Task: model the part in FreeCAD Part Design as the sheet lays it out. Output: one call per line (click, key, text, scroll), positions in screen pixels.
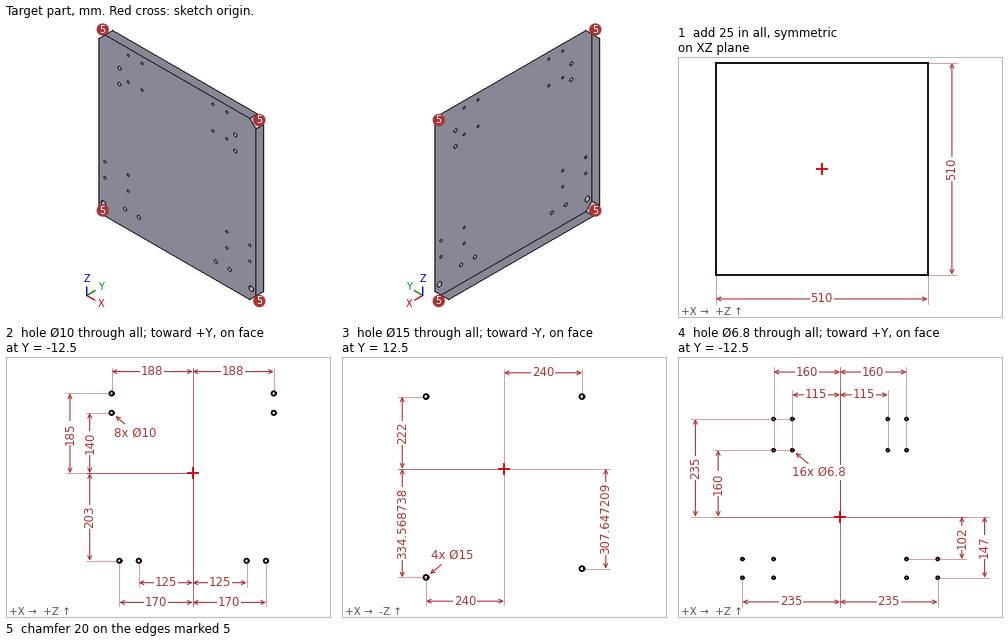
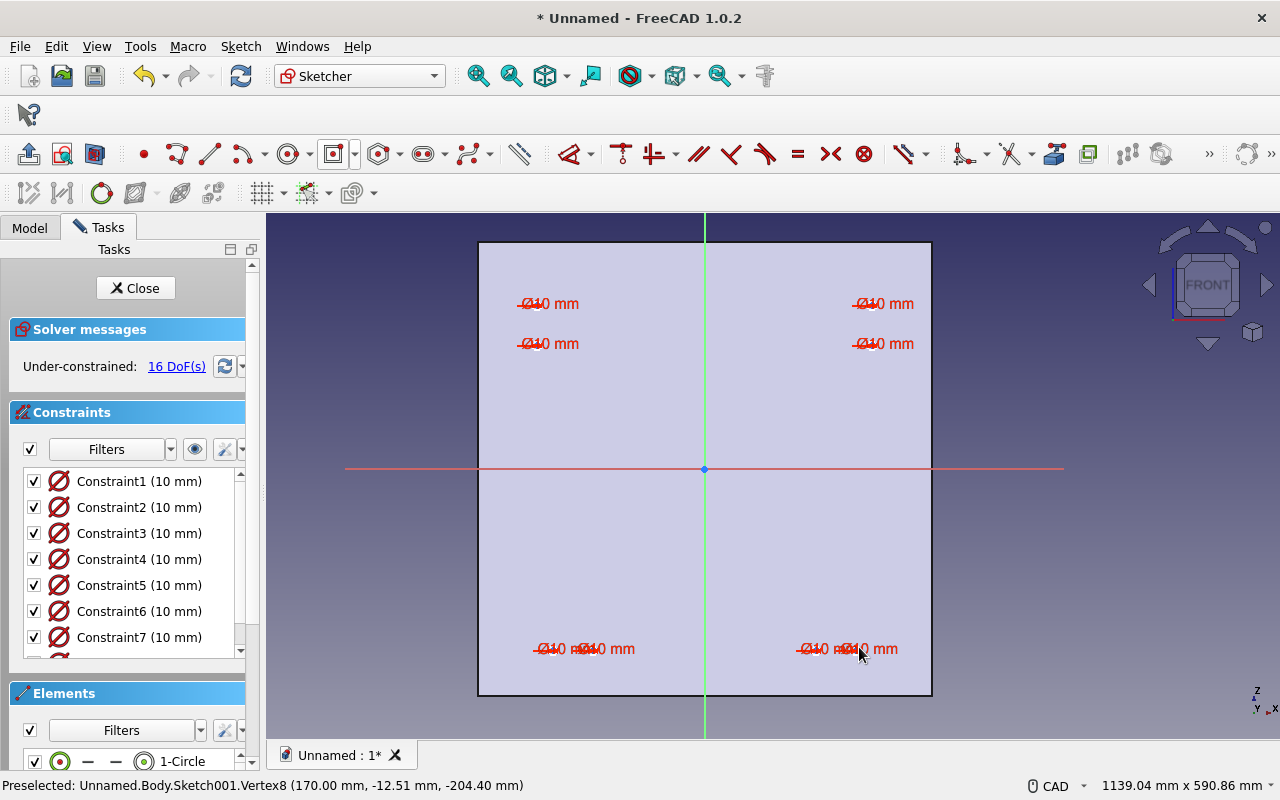
click(537, 306)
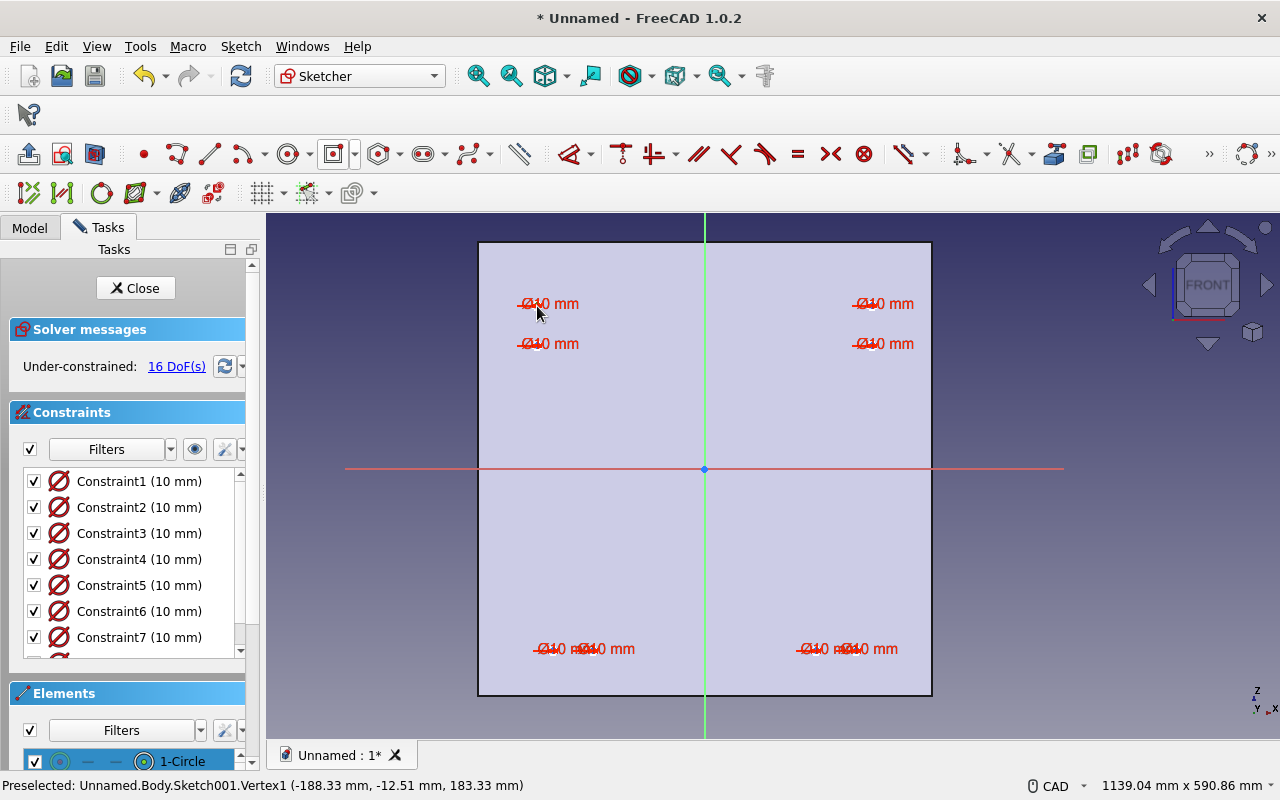
click(537, 346)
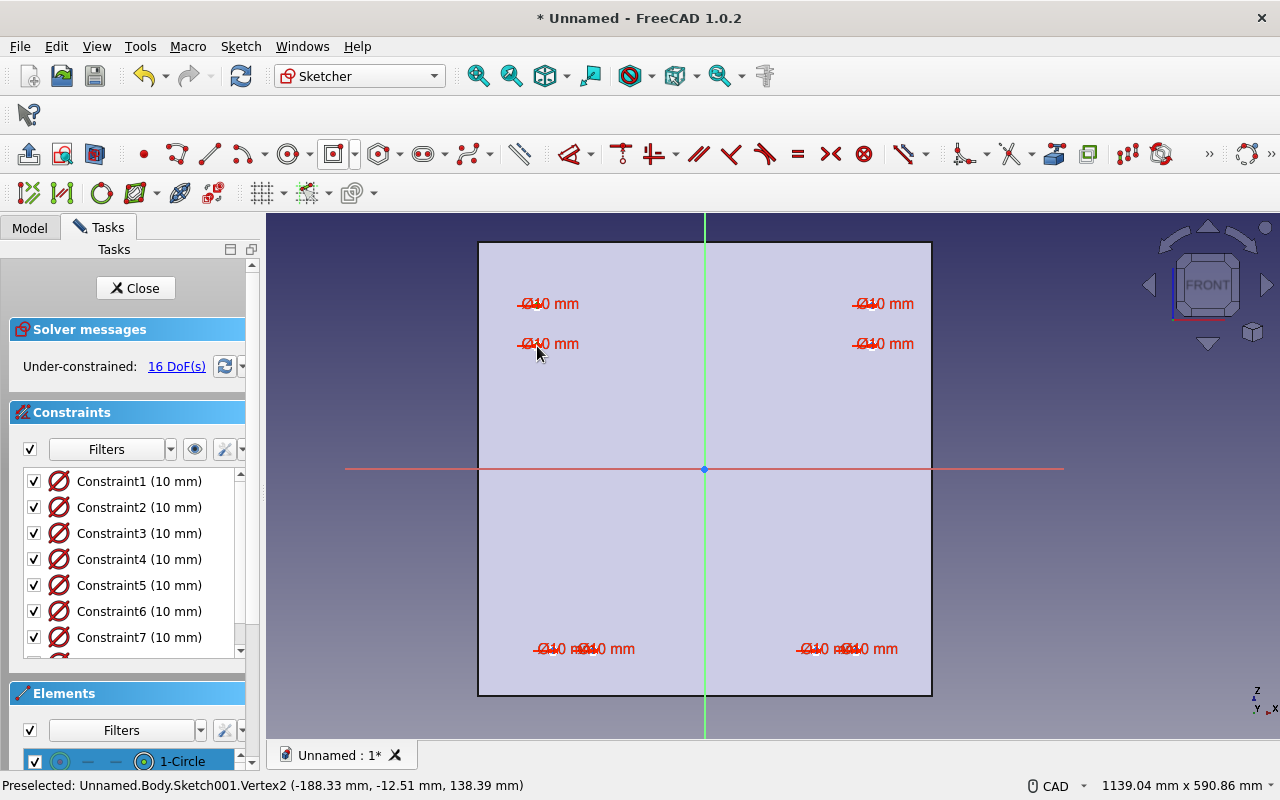
click(676, 154)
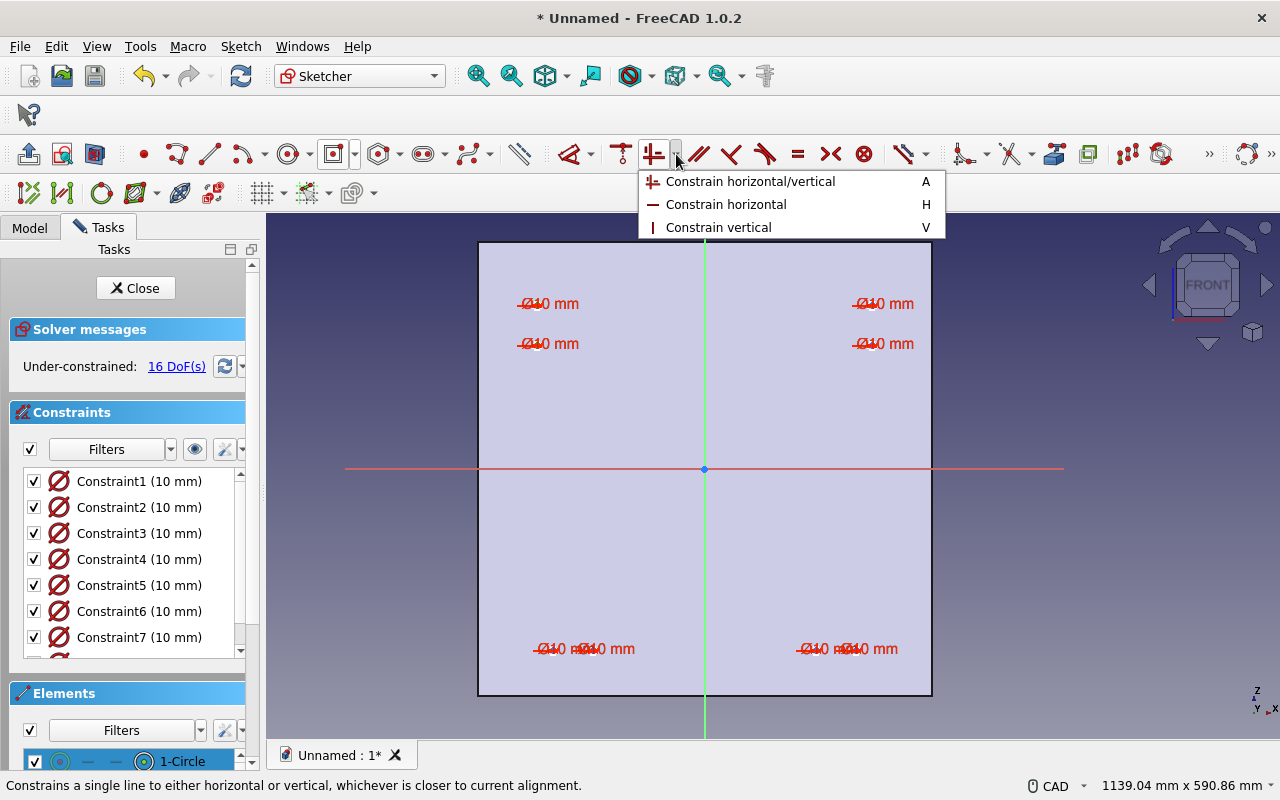
click(792, 228)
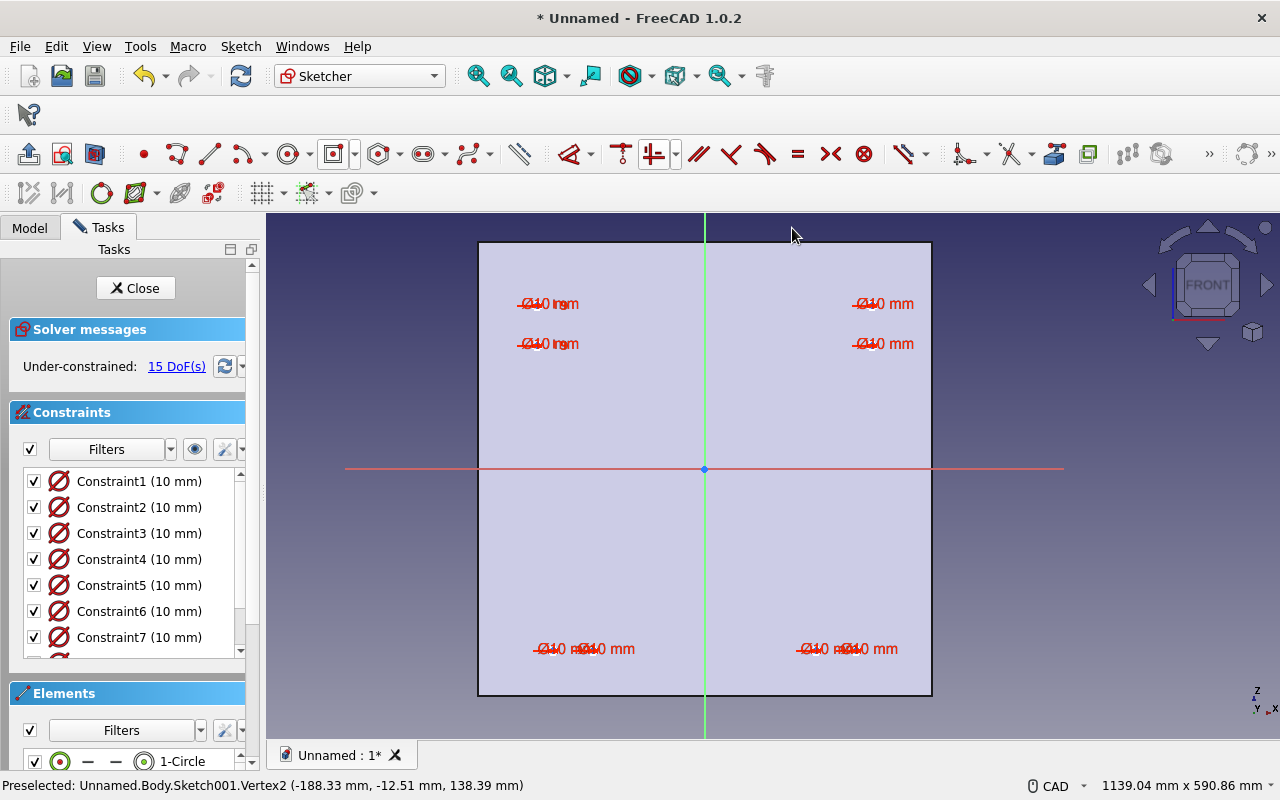
click(537, 306)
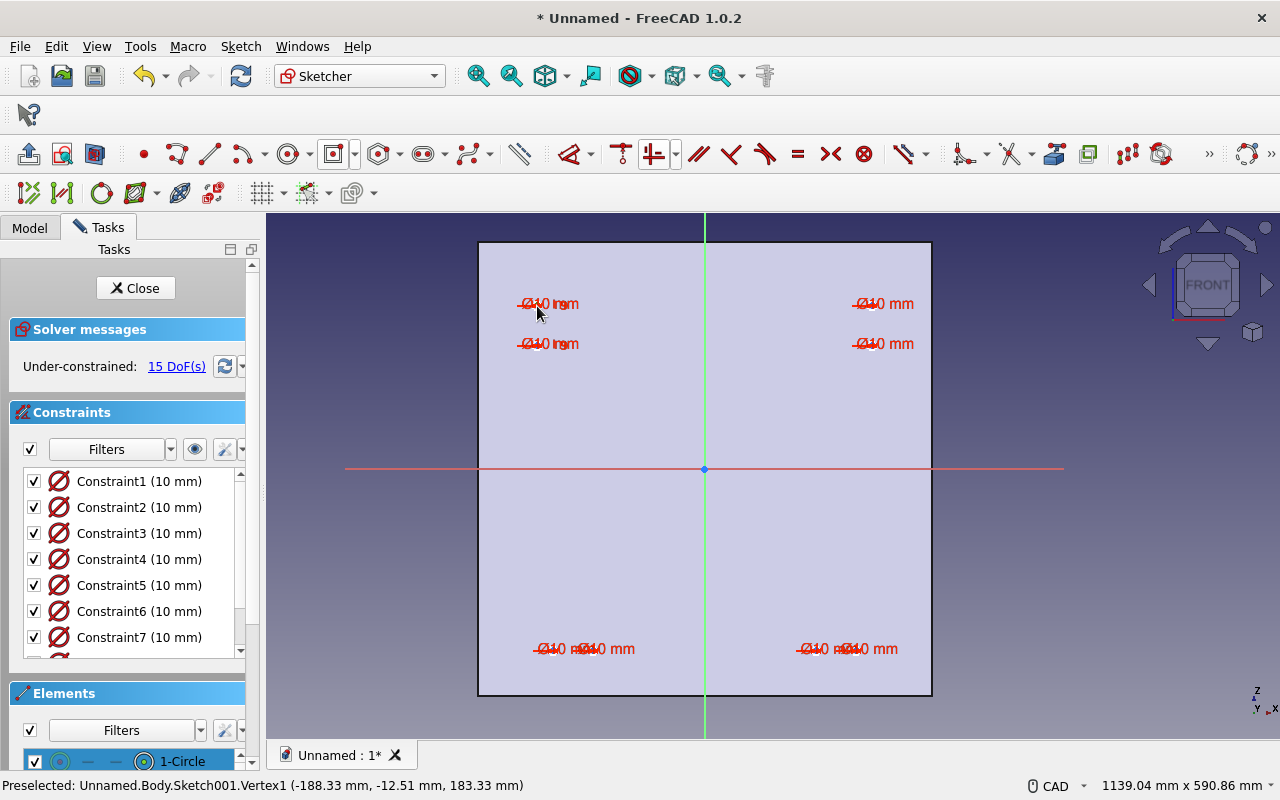
click(872, 306)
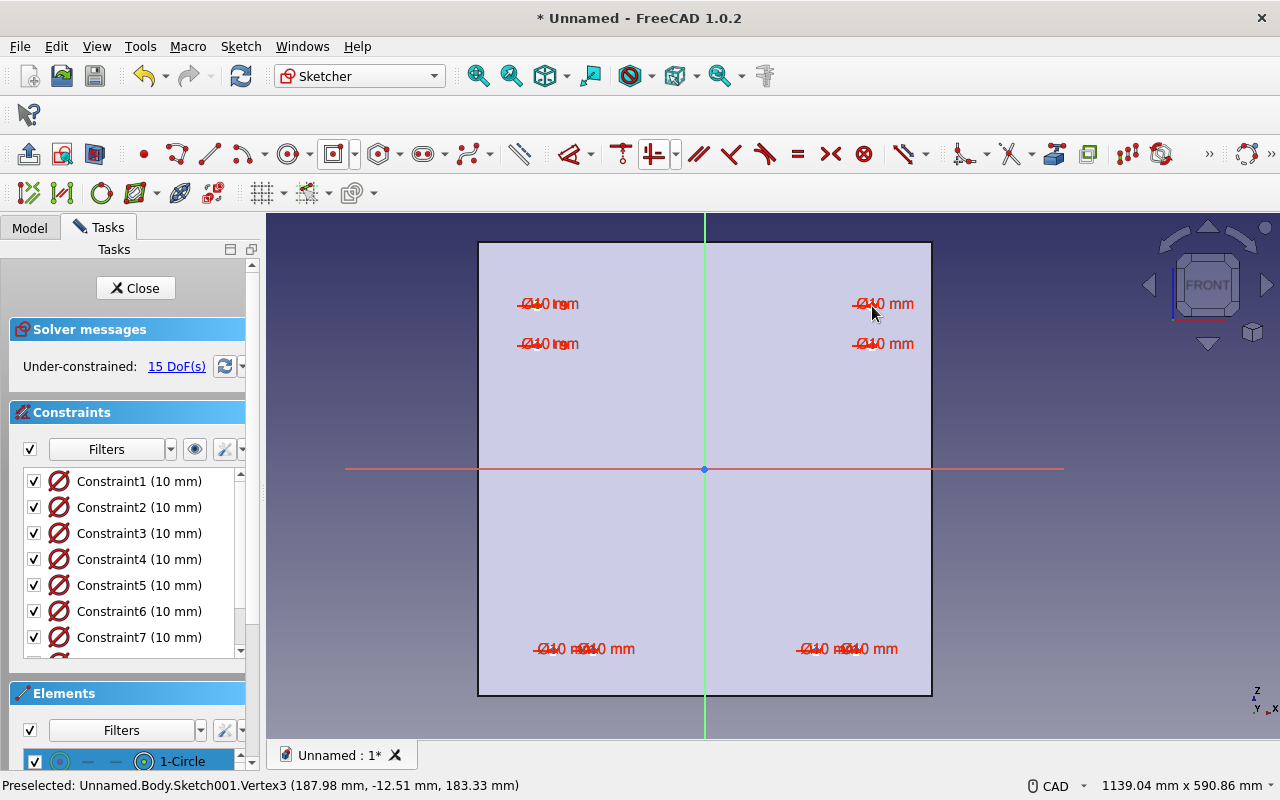
key(h)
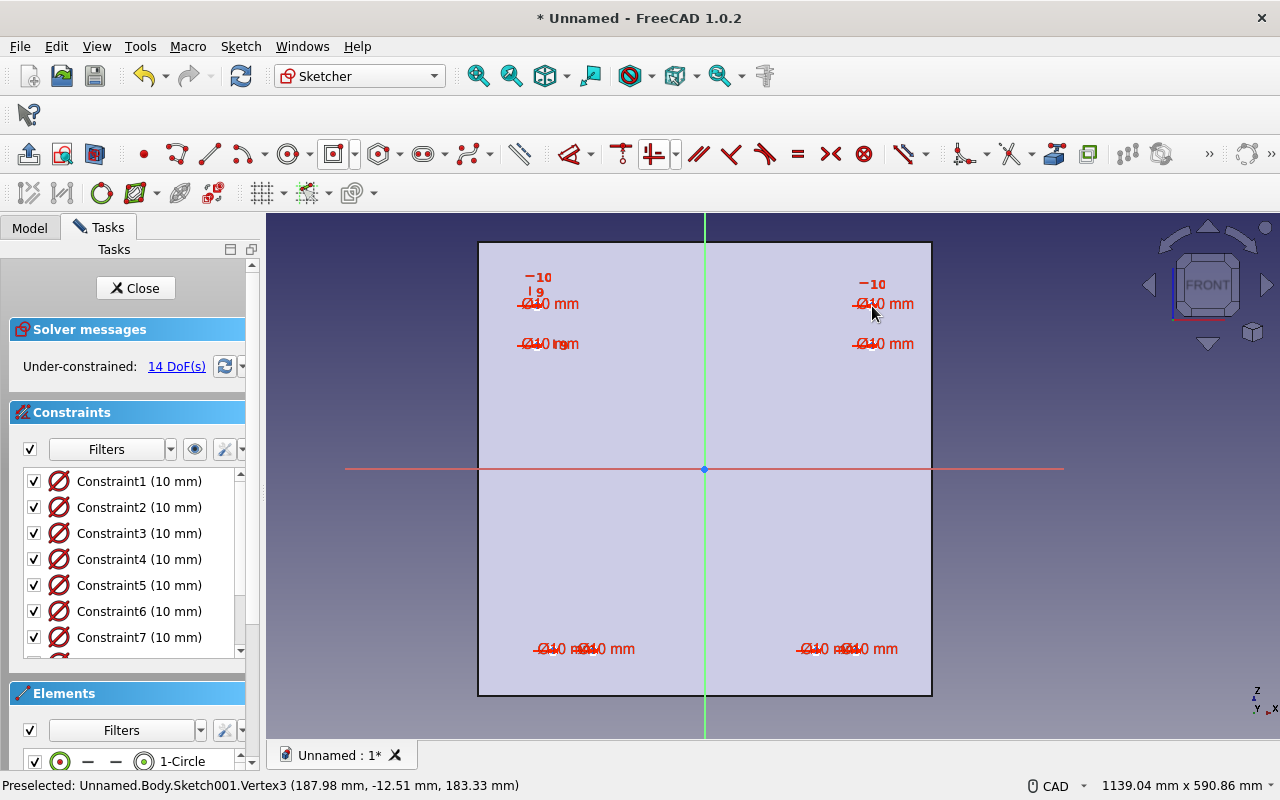
click(872, 306)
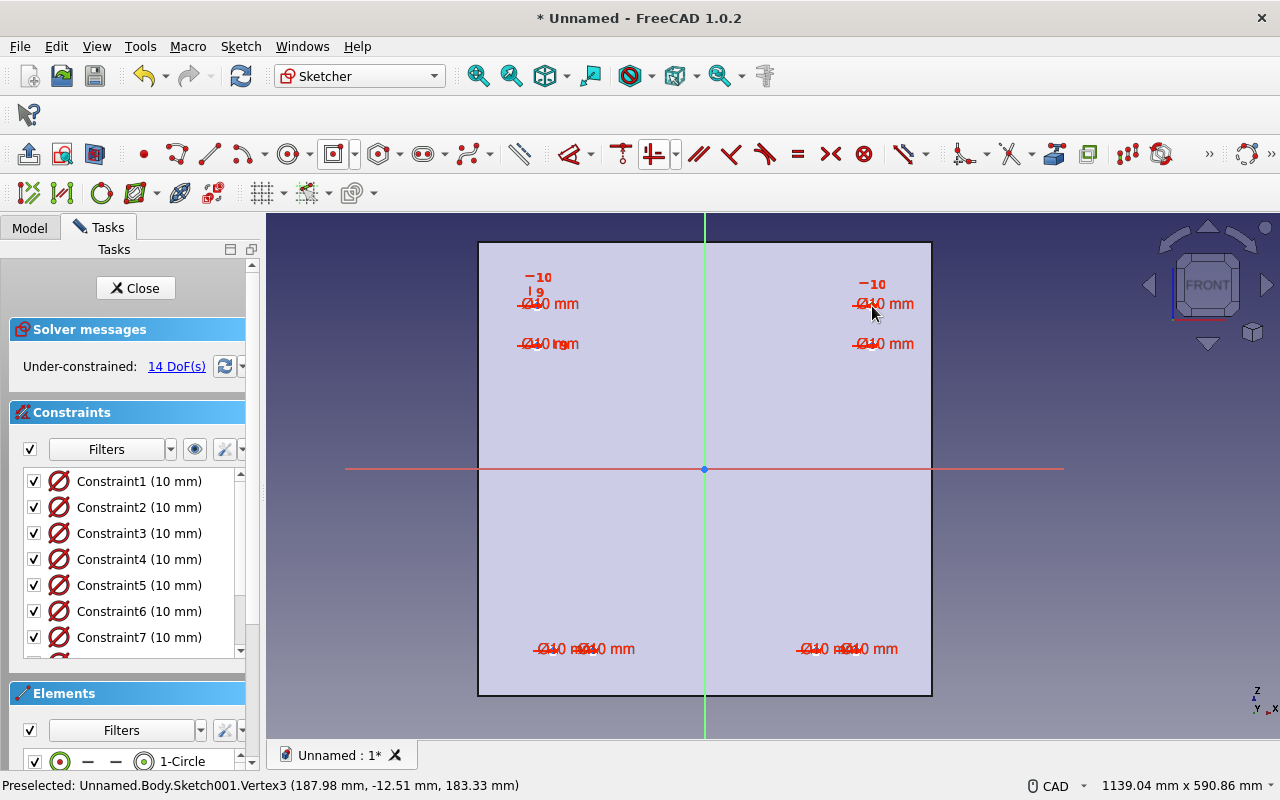
click(872, 346)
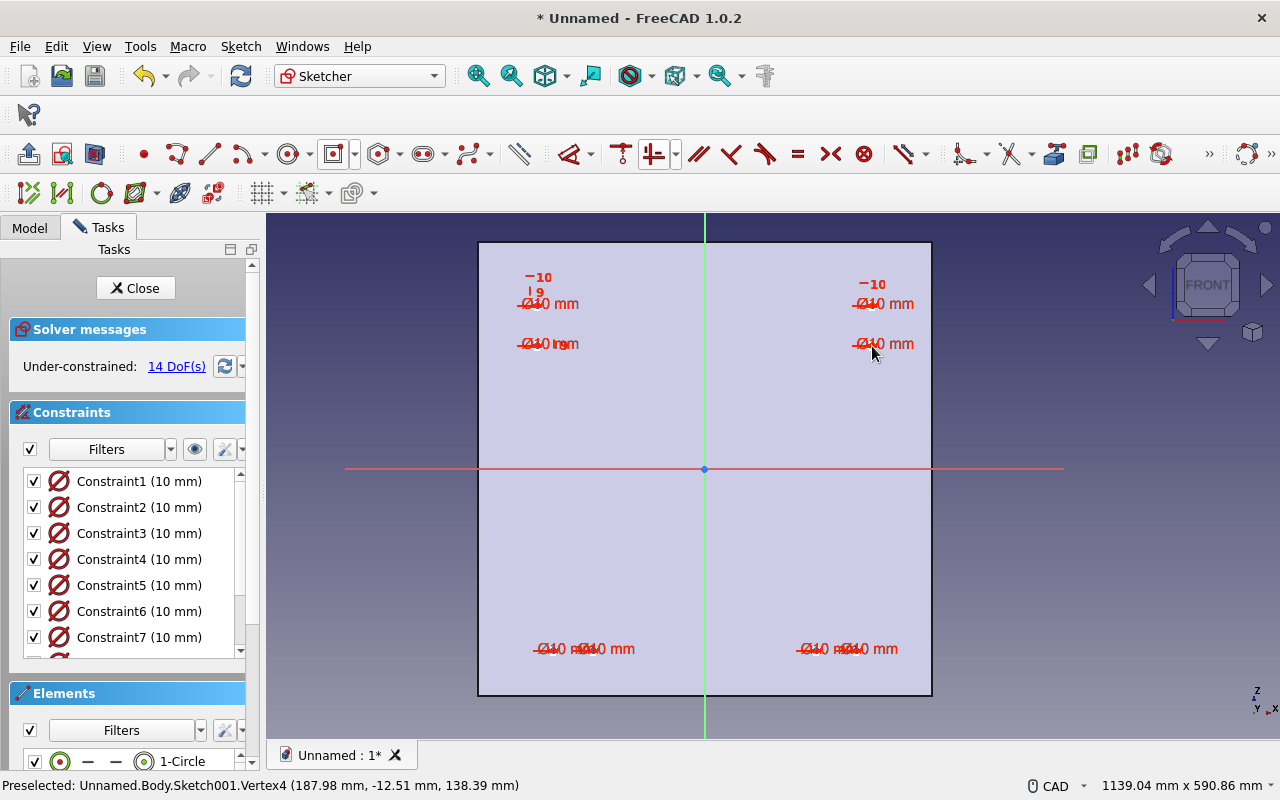
click(676, 154)